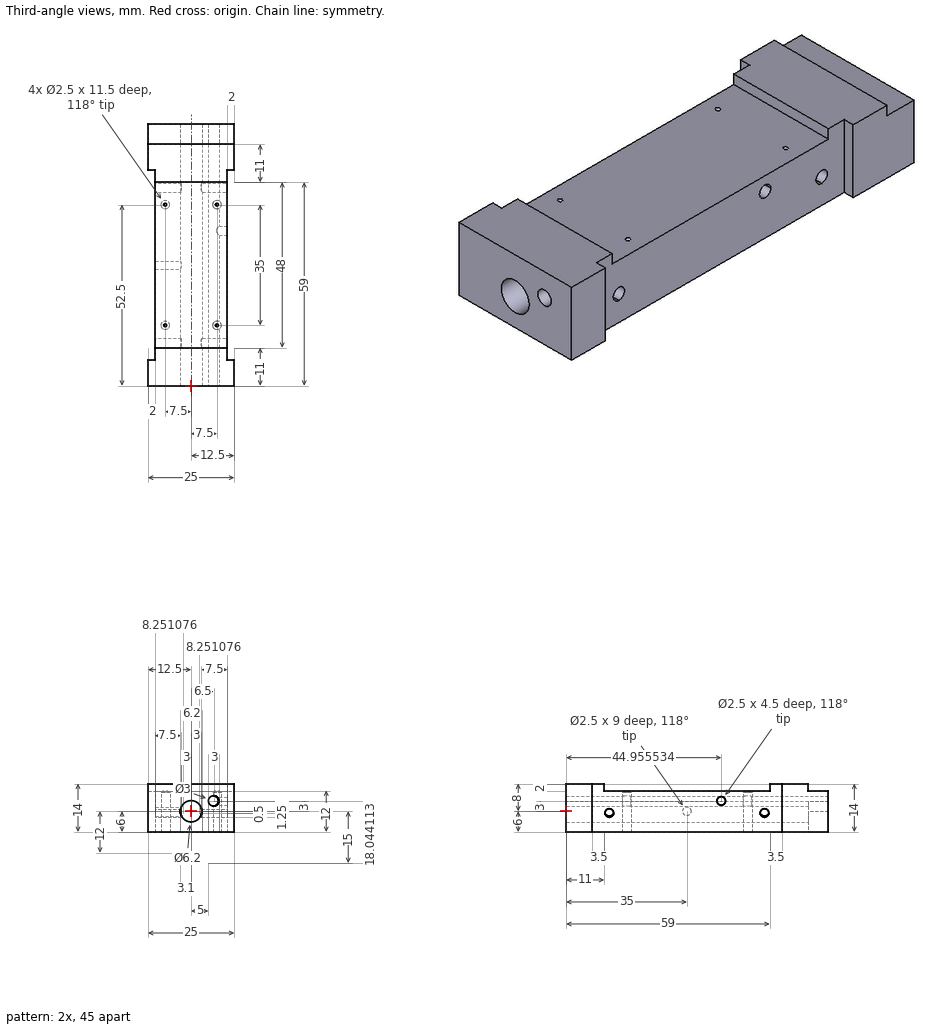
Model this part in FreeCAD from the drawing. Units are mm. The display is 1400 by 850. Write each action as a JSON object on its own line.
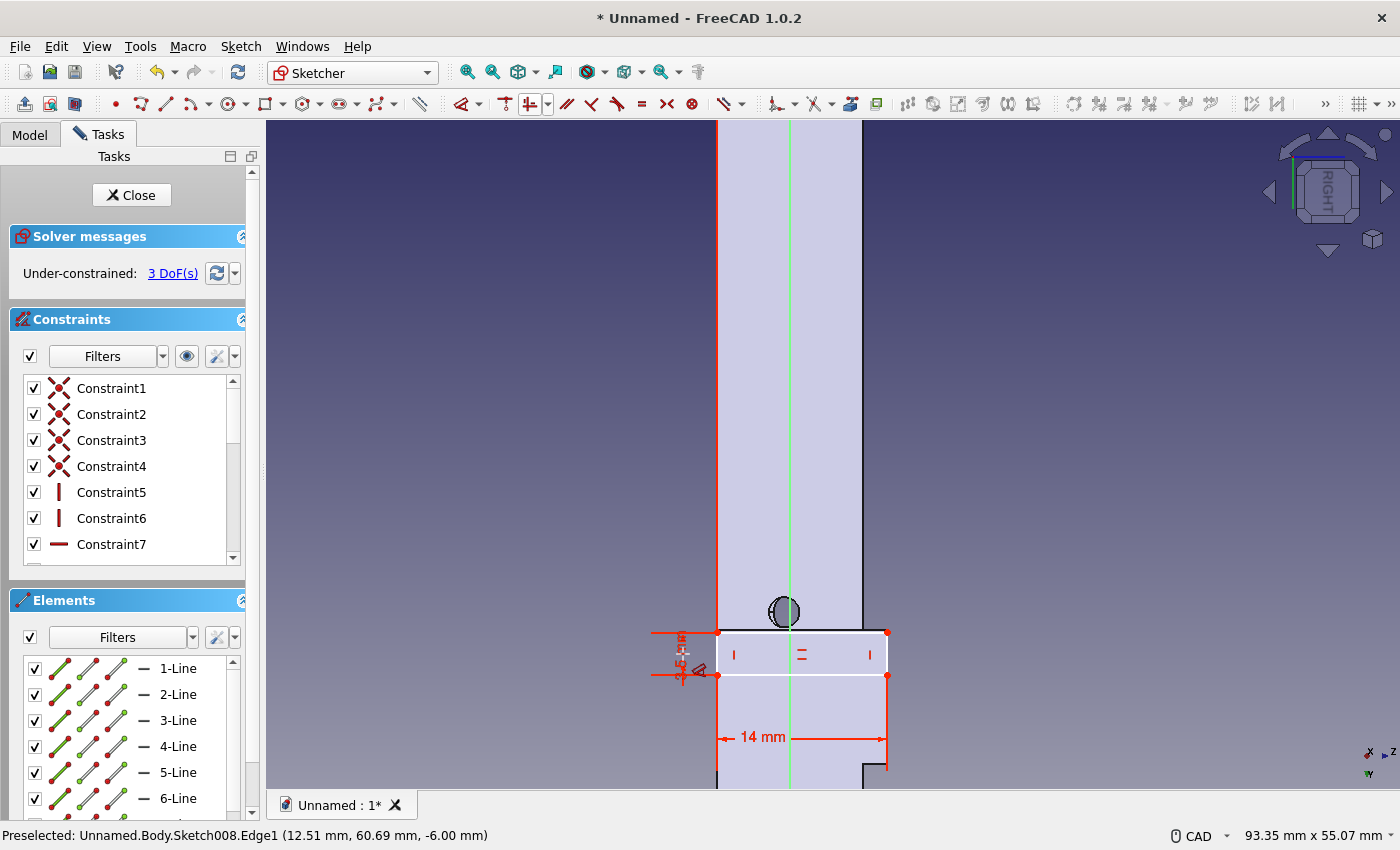
{"action": "scroll", "coordinate": [718, 650], "scroll_direction": "down", "scroll_amount": 3}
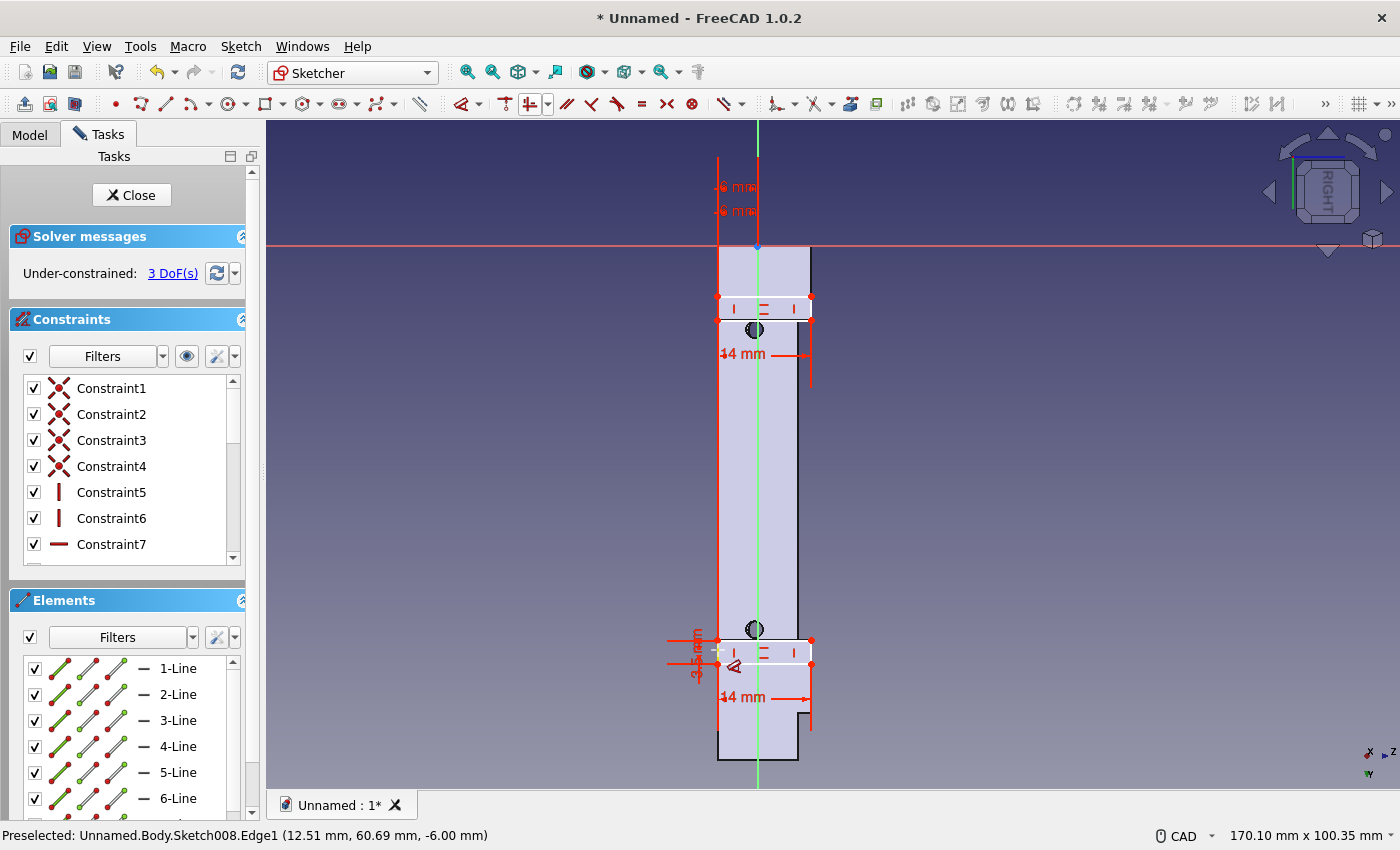
{"action": "scroll", "coordinate": [718, 304], "scroll_direction": "up", "scroll_amount": 4}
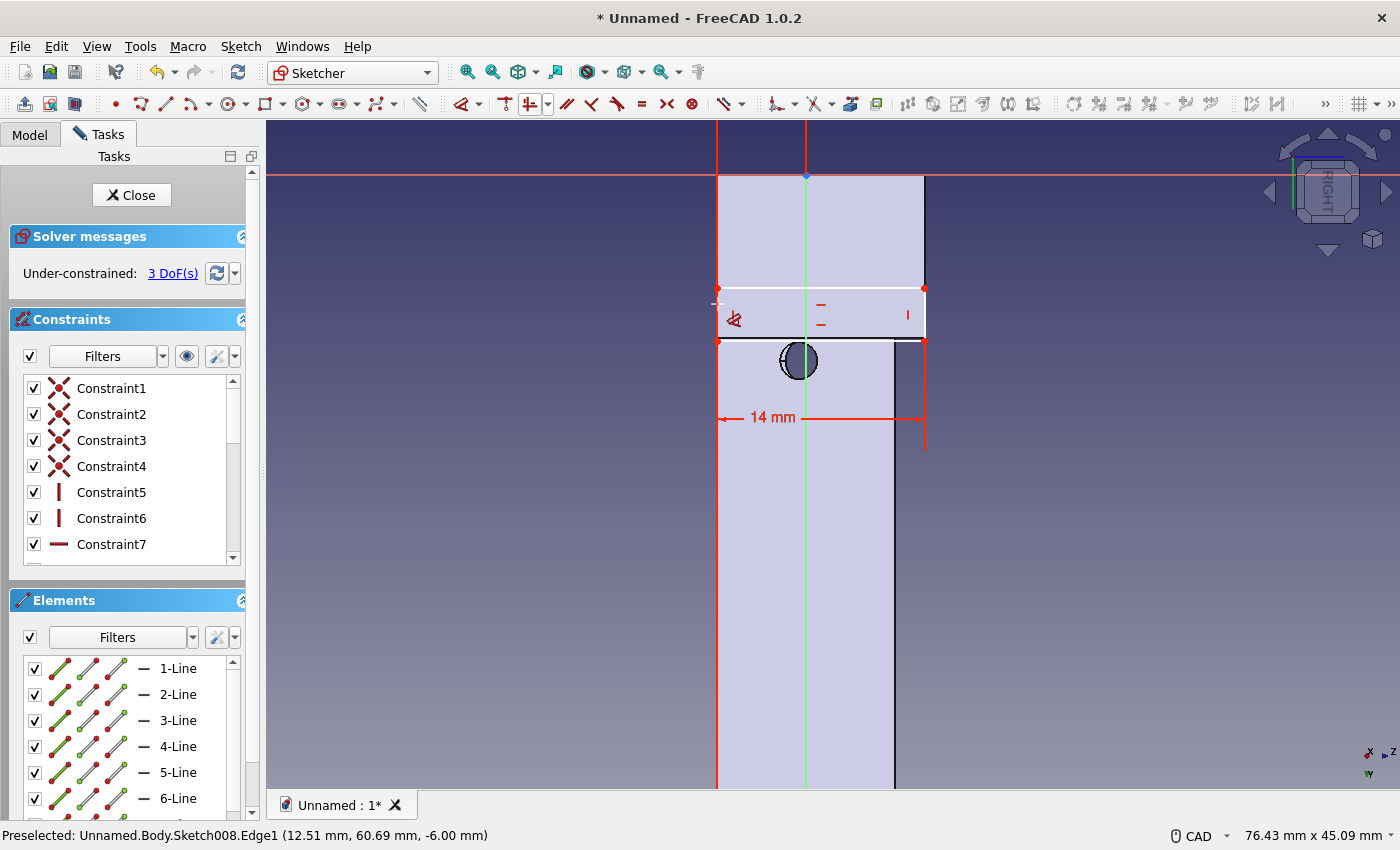
{"action": "left_click", "coordinate": [717, 304]}
{"action": "left_click", "coordinate": [683, 315]}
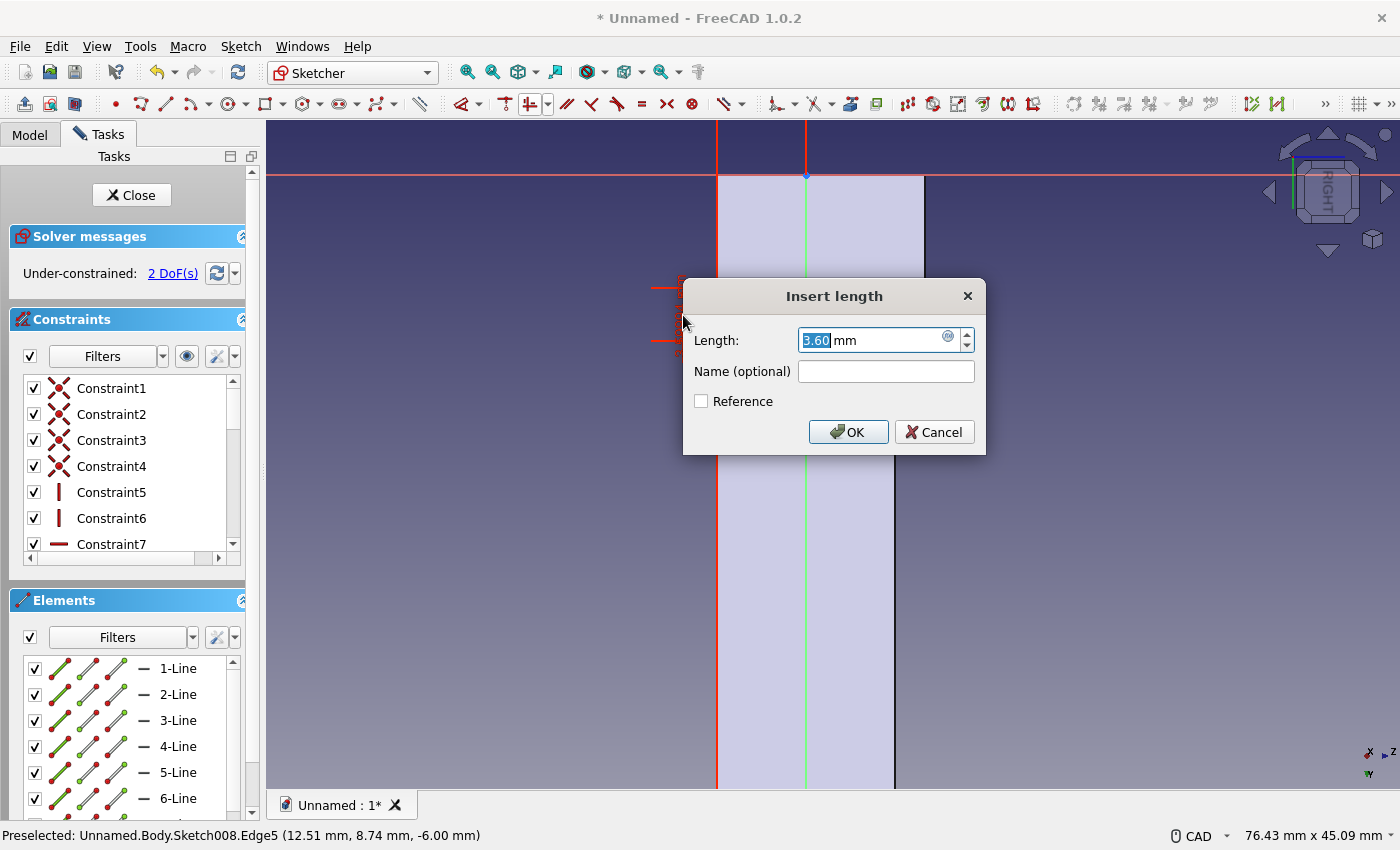
{"action": "type", "text": "3.5"}
{"action": "key", "text": "Return"}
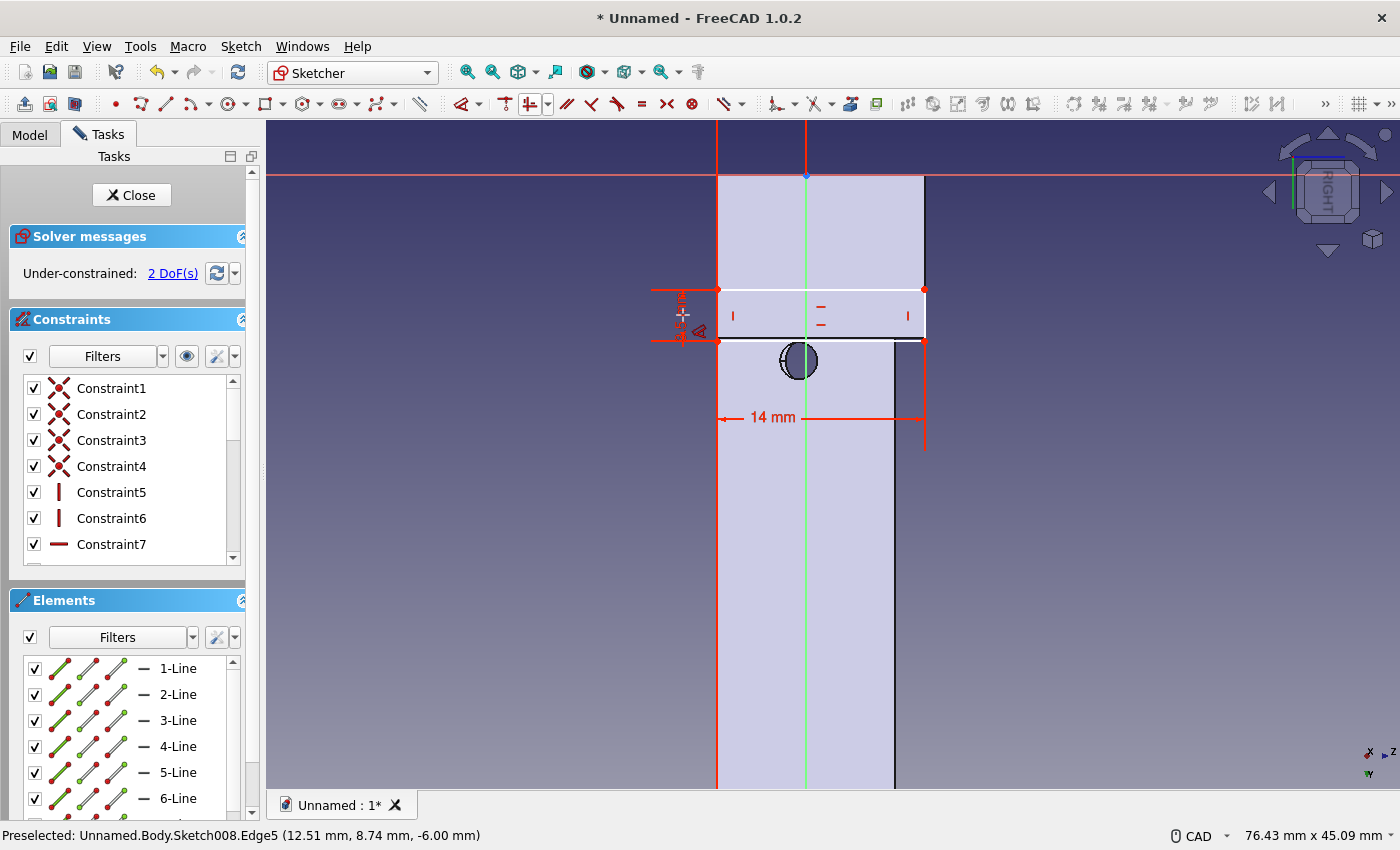
{"action": "scroll", "coordinate": [718, 304], "scroll_direction": "down", "scroll_amount": 4}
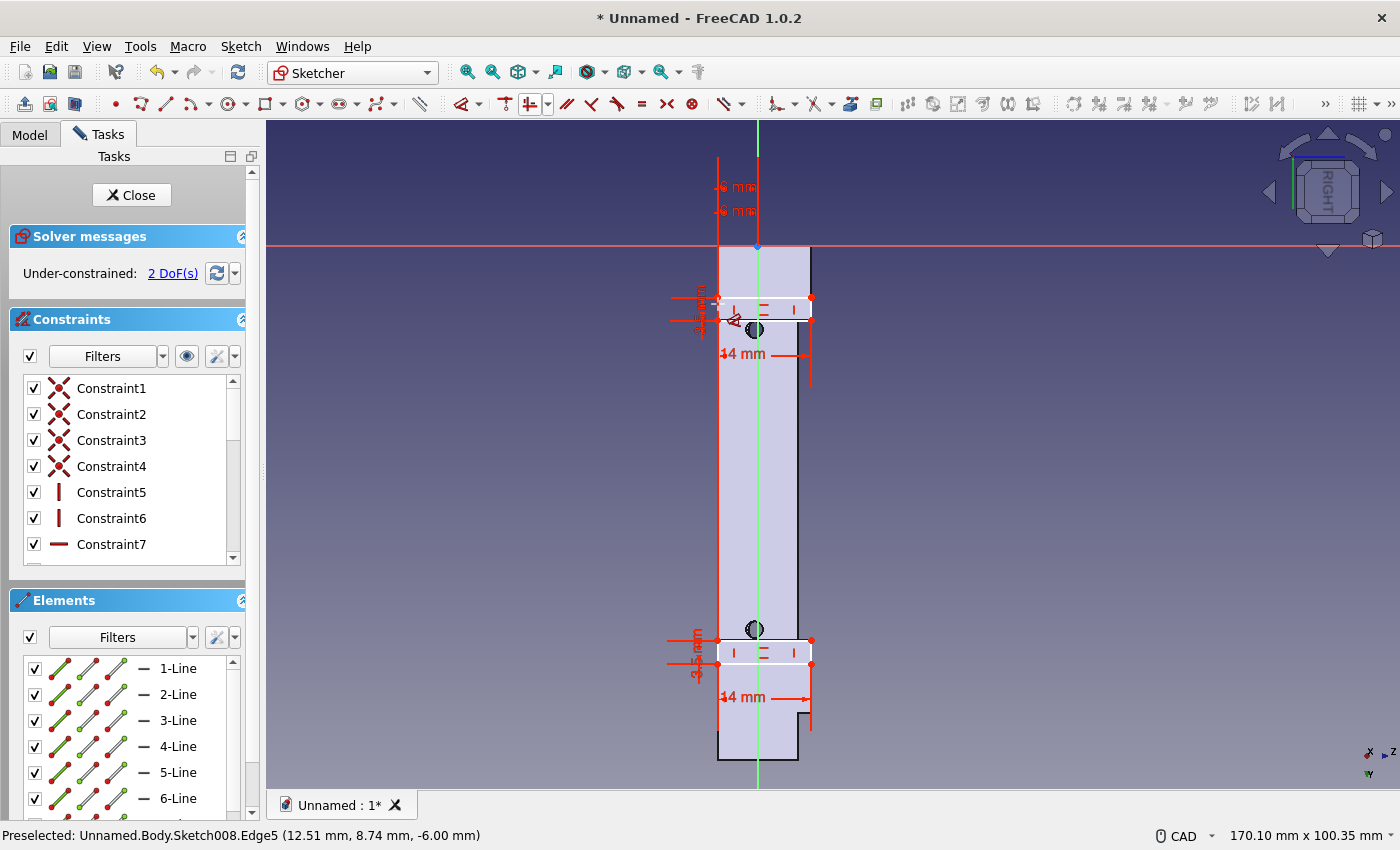
{"action": "left_click", "coordinate": [718, 641]}
{"action": "left_click", "coordinate": [684, 444]}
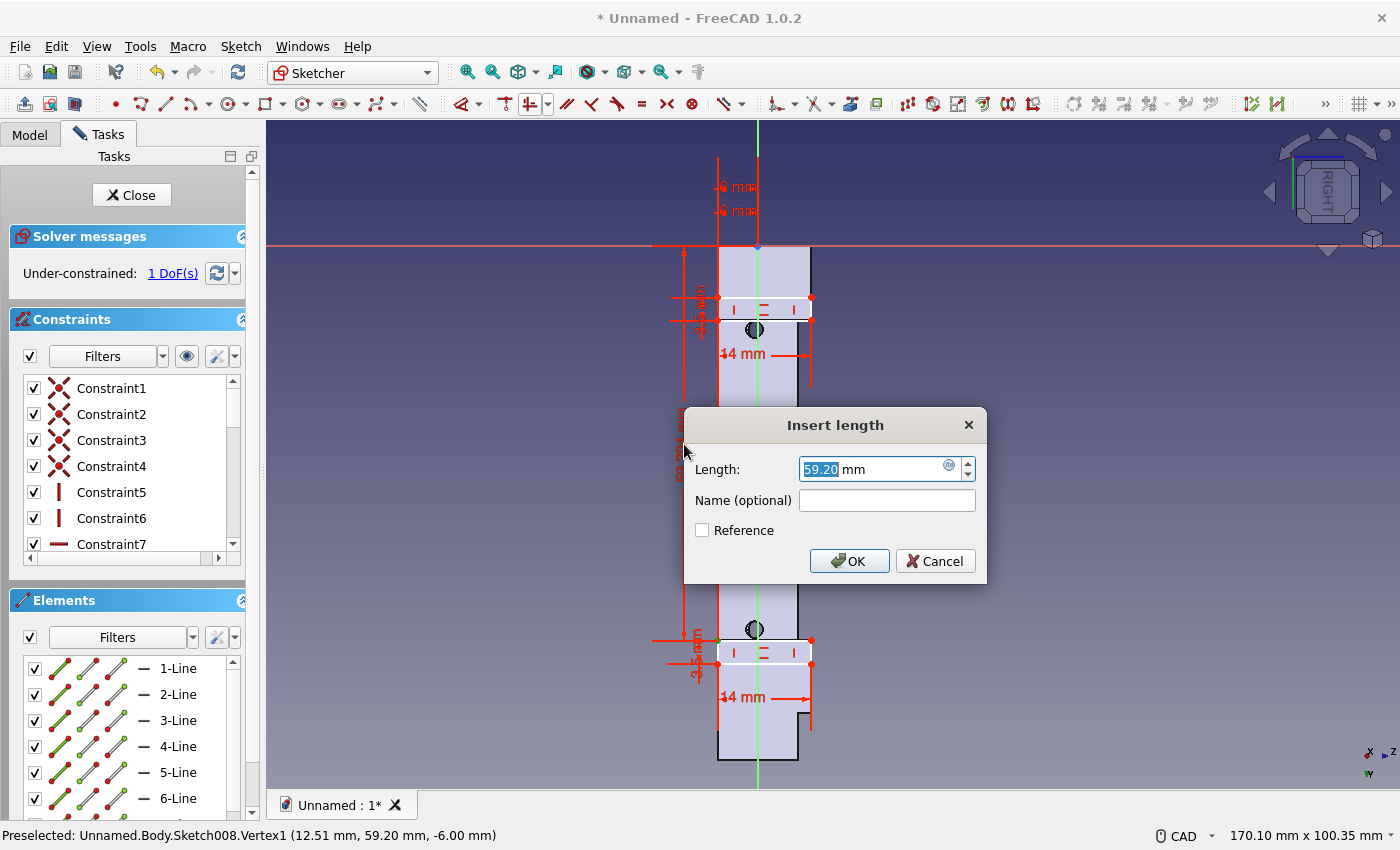
{"action": "type", "text": "59"}
{"action": "key", "text": "Return"}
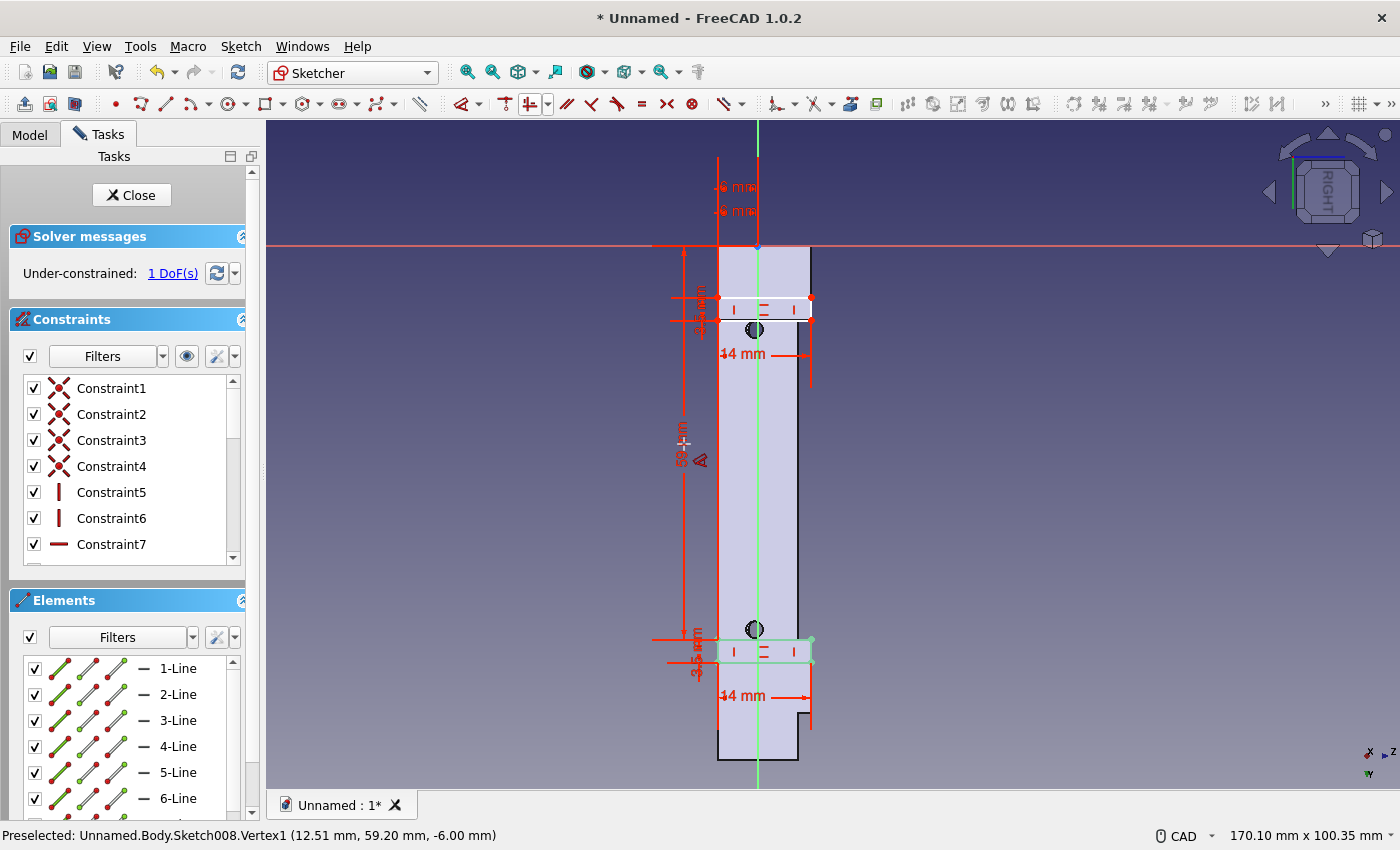
{"action": "left_click", "coordinate": [718, 321]}
{"action": "left_click", "coordinate": [684, 284]}